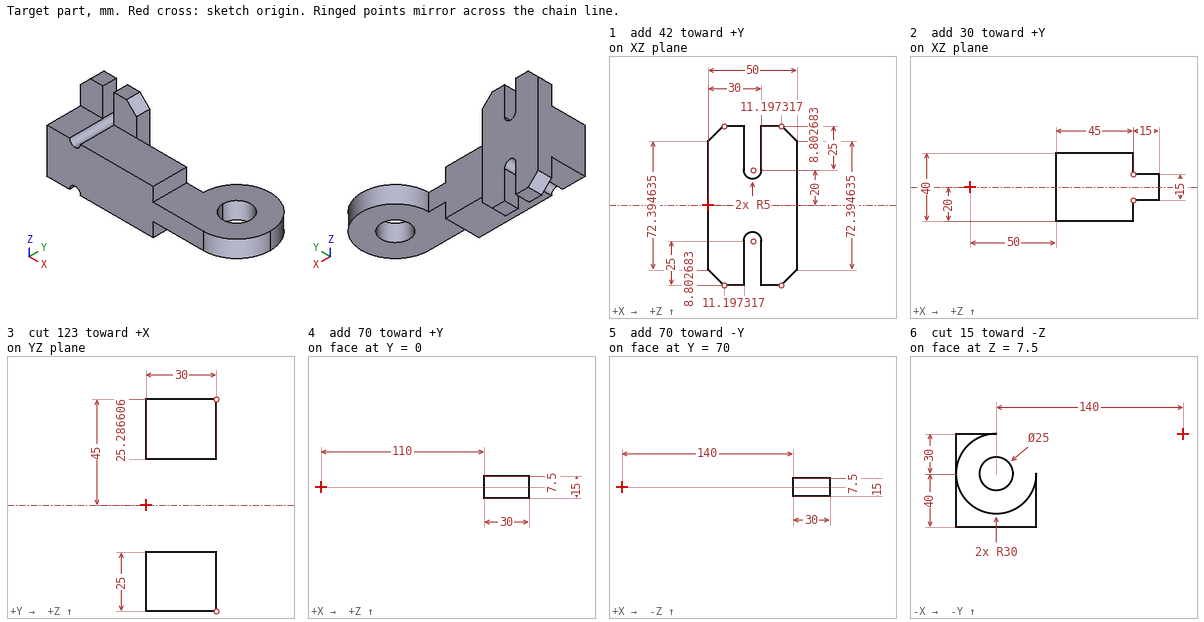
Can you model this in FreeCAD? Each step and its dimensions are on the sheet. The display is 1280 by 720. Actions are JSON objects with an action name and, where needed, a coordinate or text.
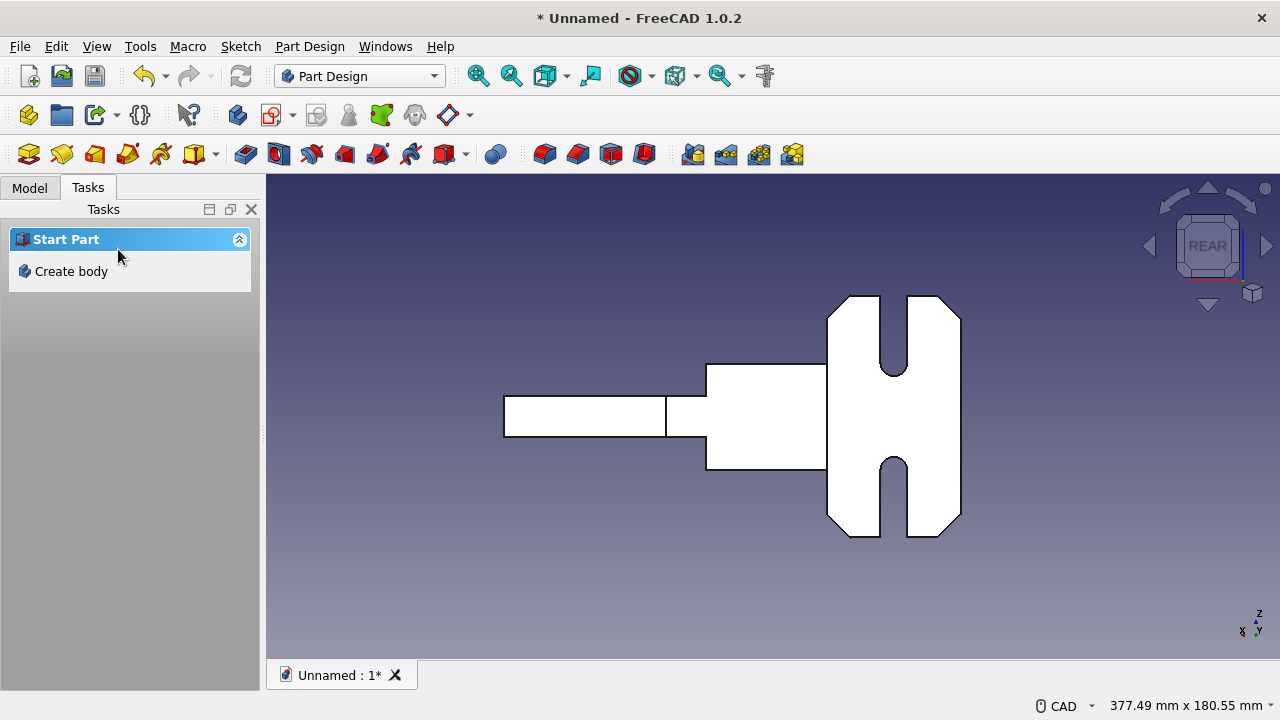
{"action": "key", "text": "0"}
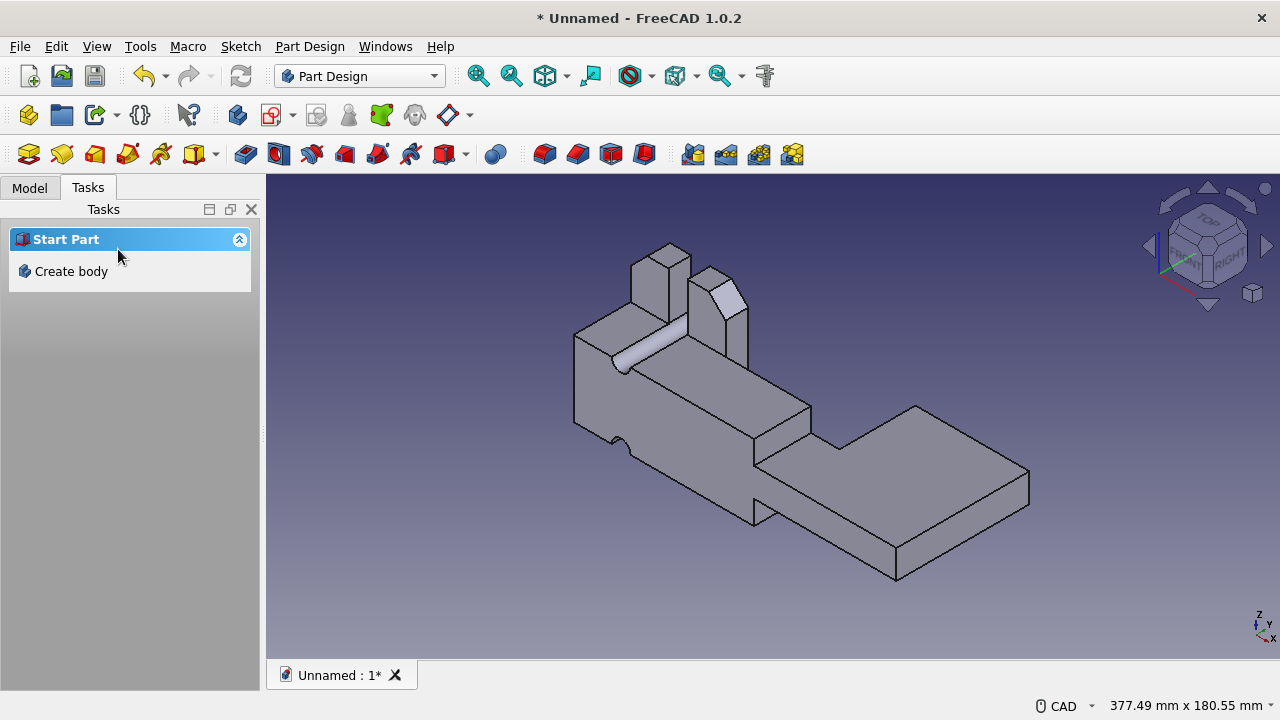
{"action": "left_click", "coordinate": [479, 76]}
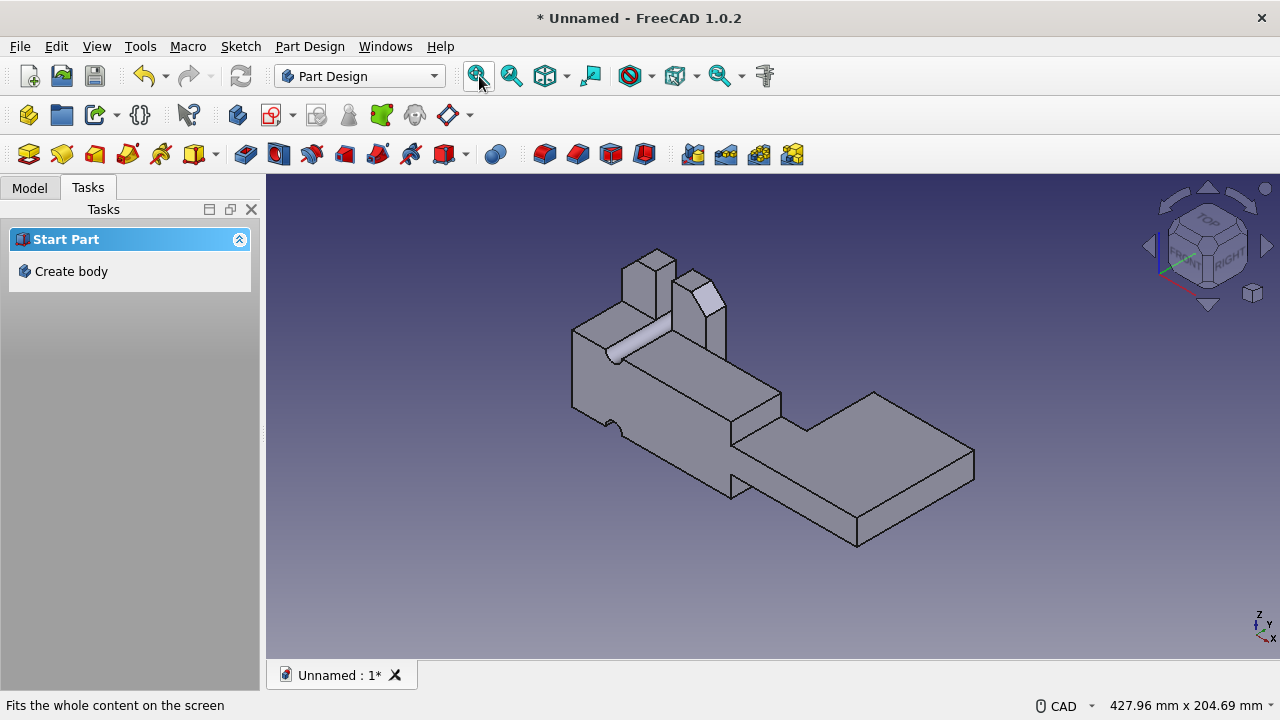
{"action": "left_click", "coordinate": [871, 457]}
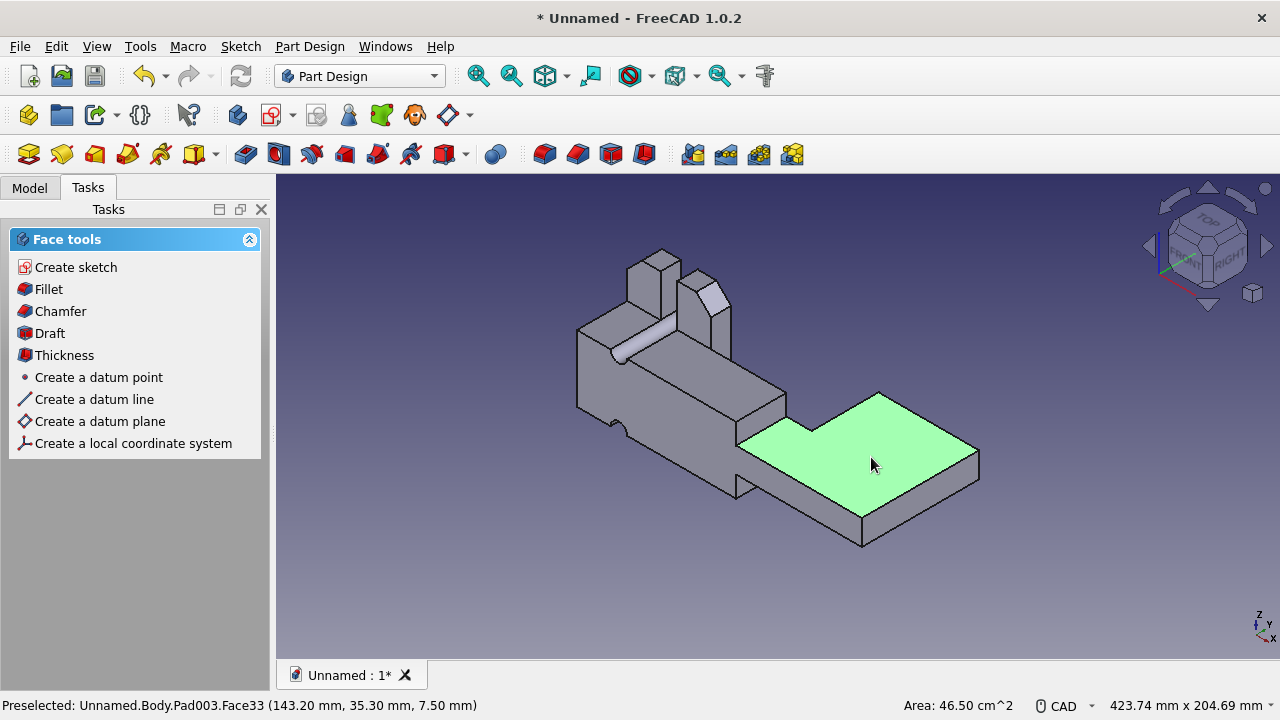
{"action": "left_click", "coordinate": [270, 116]}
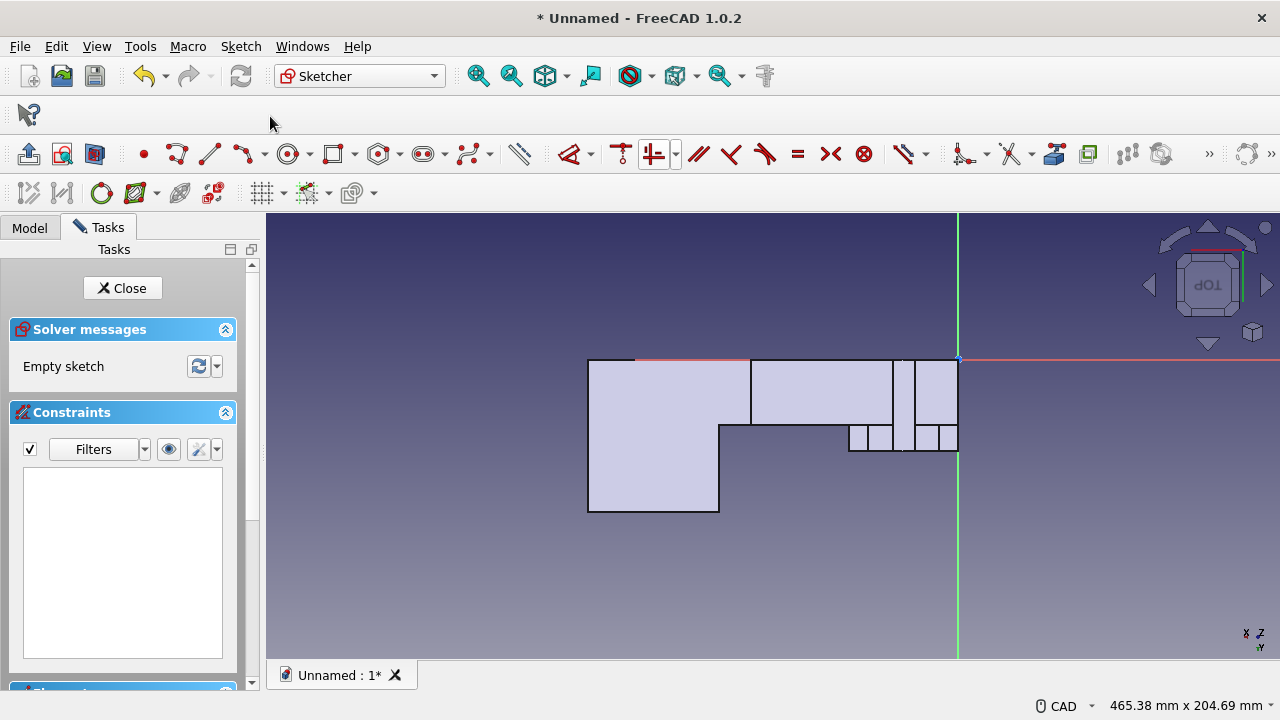
{"action": "left_click", "coordinate": [95, 154]}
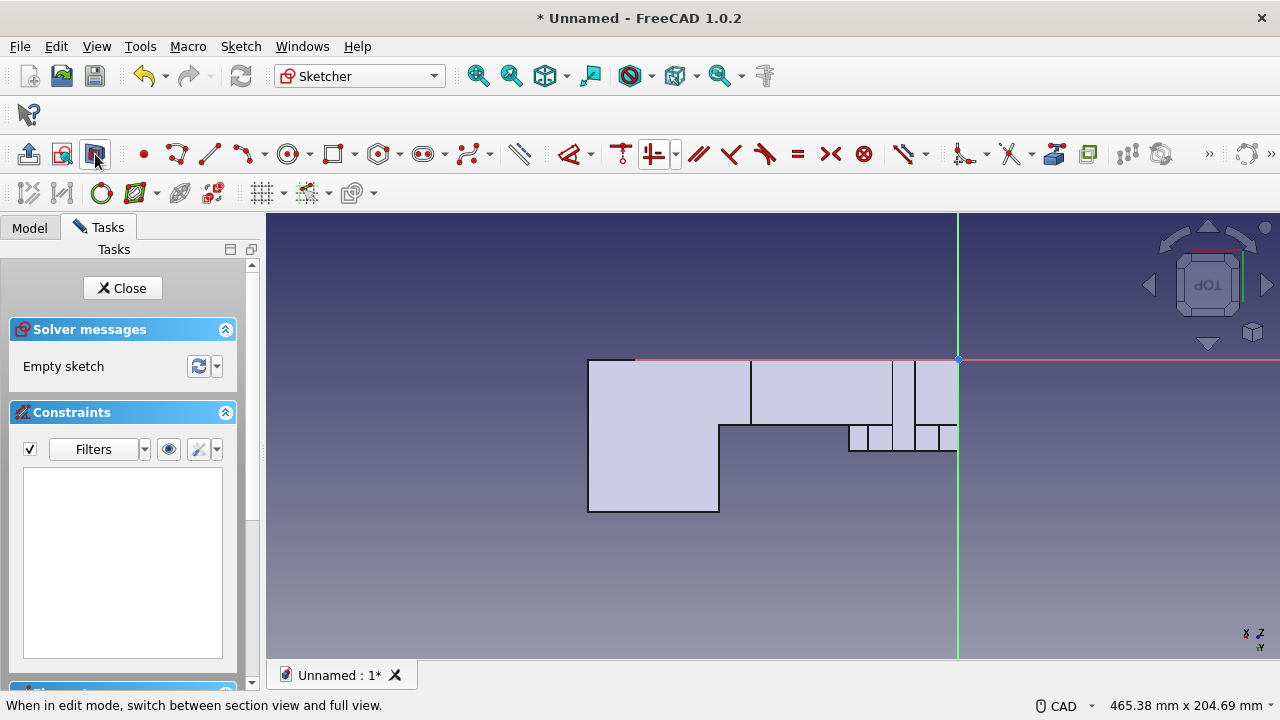
{"action": "scroll", "coordinate": [912, 436], "scroll_direction": "up", "scroll_amount": 2}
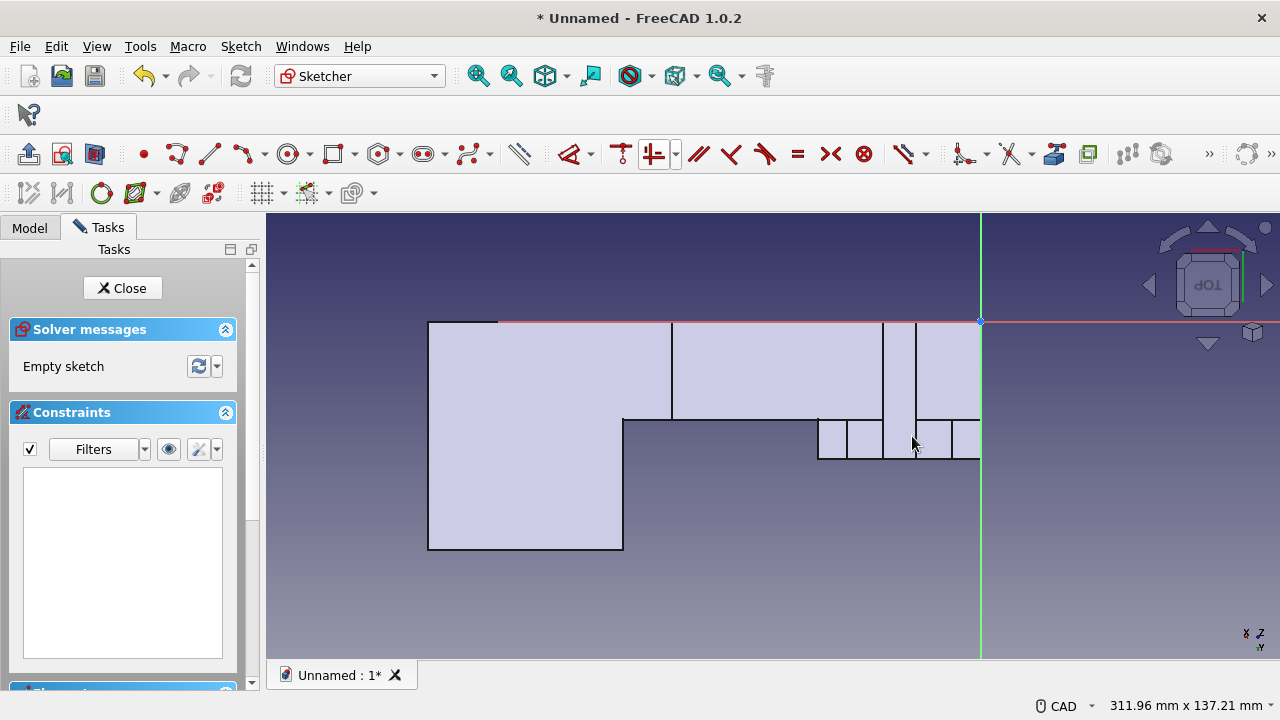
{"action": "key", "text": "g m"}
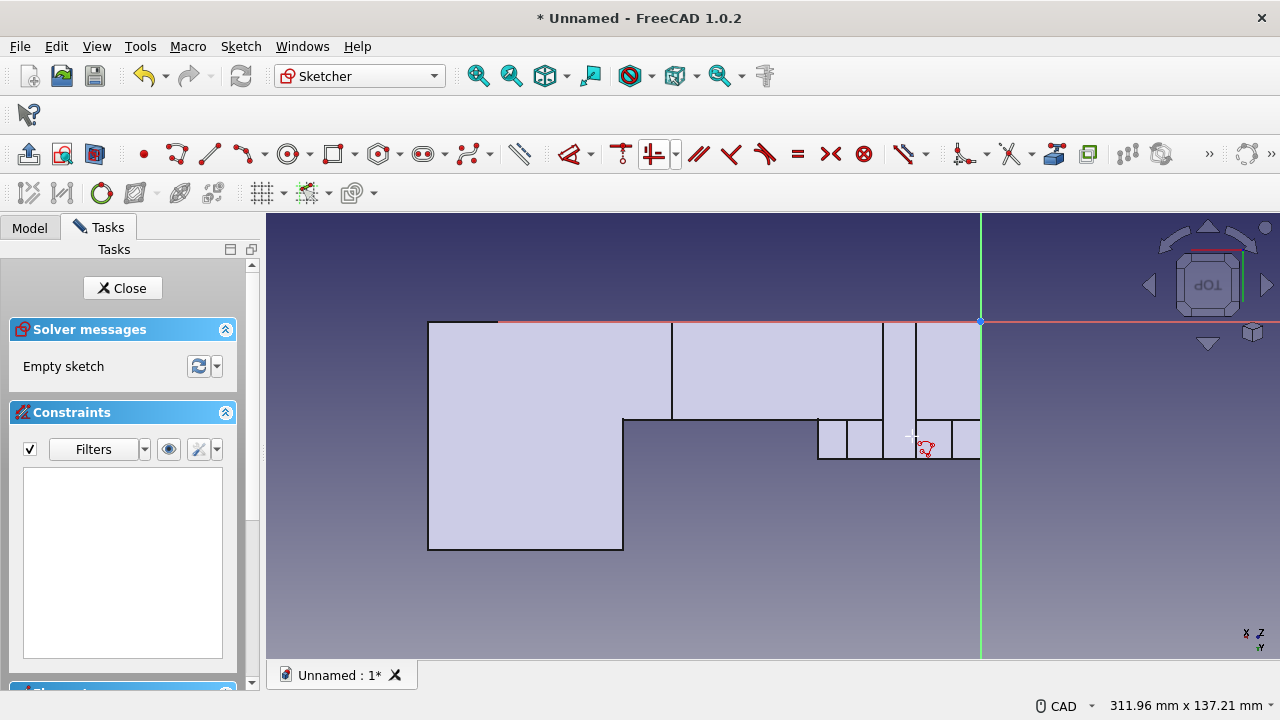
{"action": "left_click", "coordinate": [428, 420]}
{"action": "left_click", "coordinate": [428, 550]}
{"action": "left_click", "coordinate": [623, 550]}
{"action": "left_click", "coordinate": [623, 420]}
{"action": "right_click", "coordinate": [623, 420]}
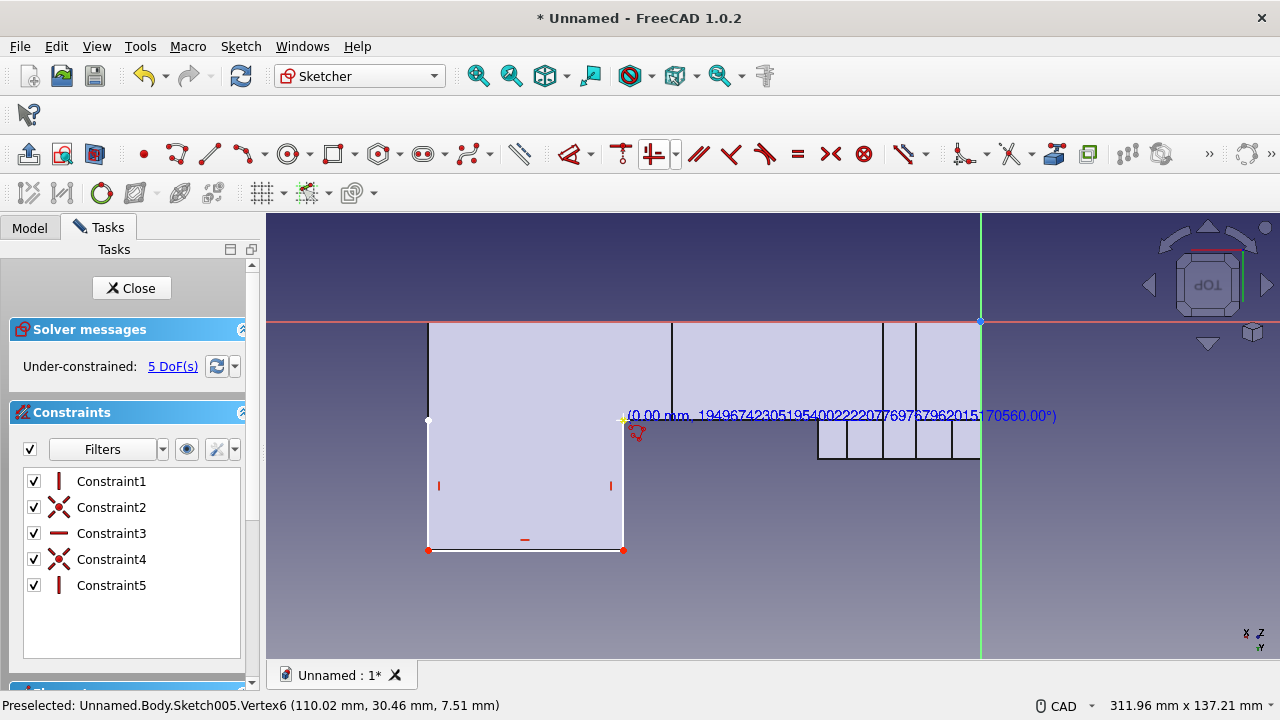
{"action": "left_click", "coordinate": [242, 154]}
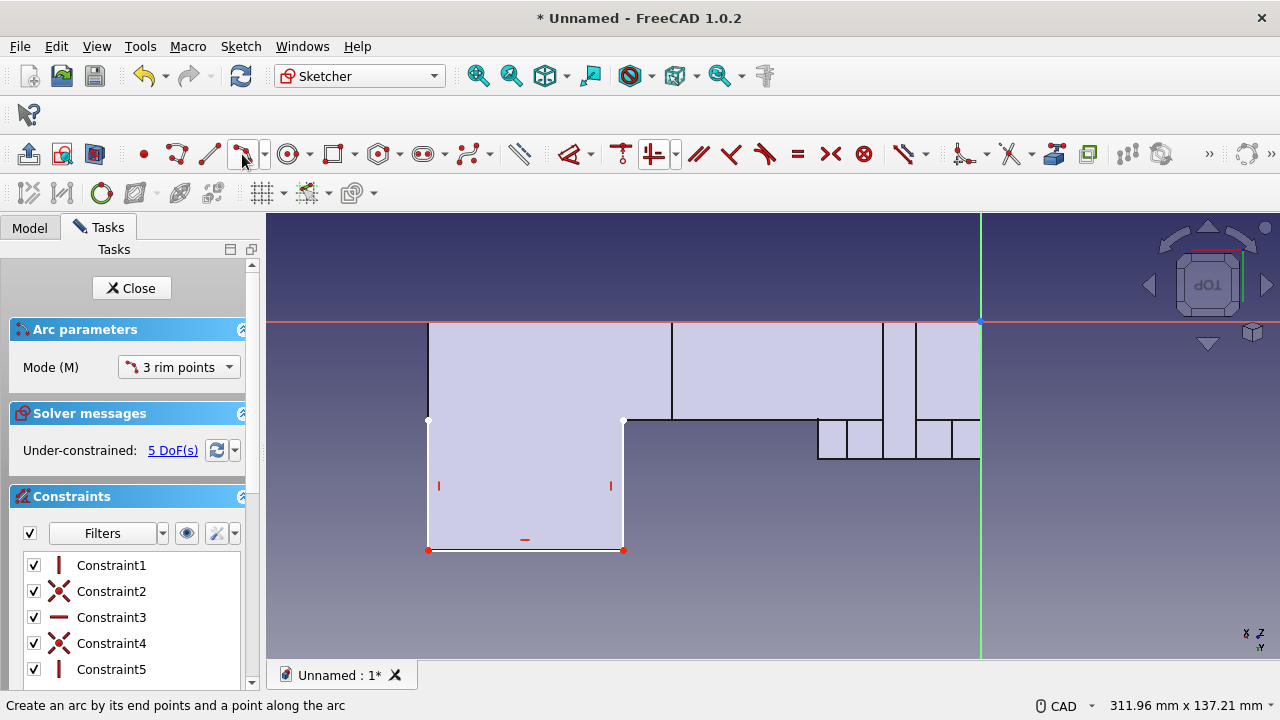
{"action": "left_click", "coordinate": [623, 421]}
{"action": "left_click", "coordinate": [428, 421]}
{"action": "left_click", "coordinate": [526, 517]}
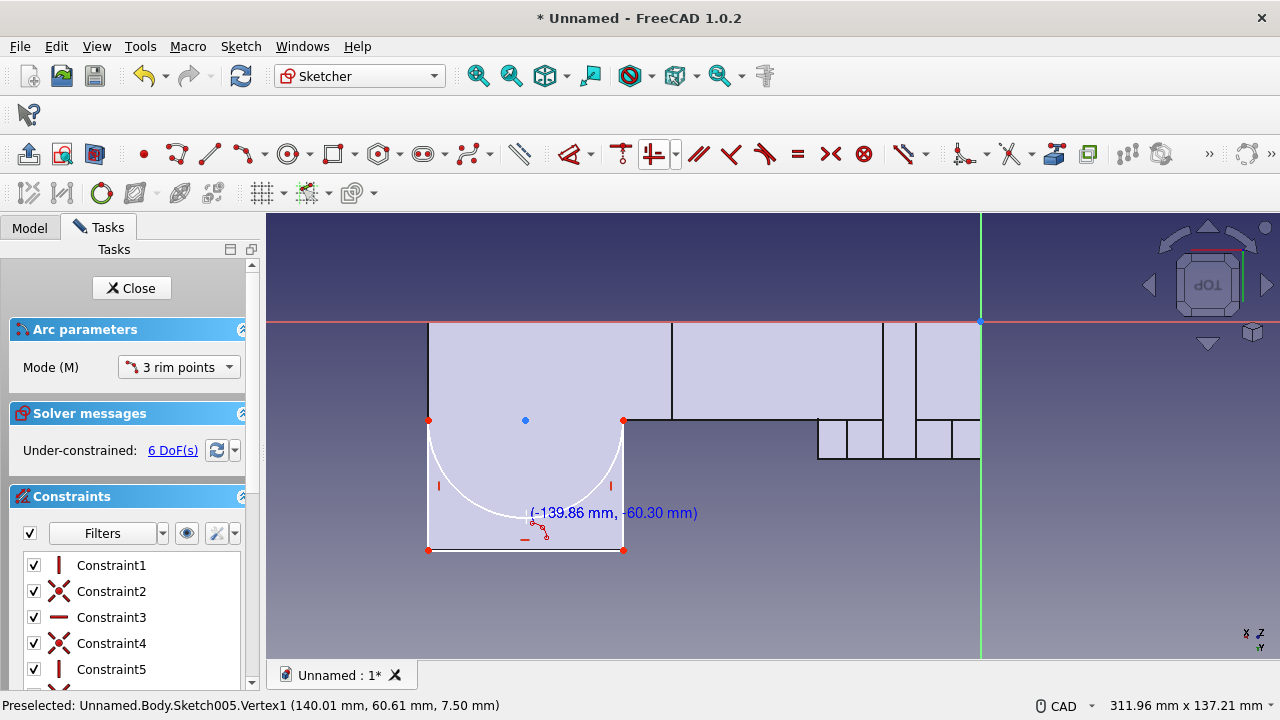
{"action": "key", "text": "g m"}